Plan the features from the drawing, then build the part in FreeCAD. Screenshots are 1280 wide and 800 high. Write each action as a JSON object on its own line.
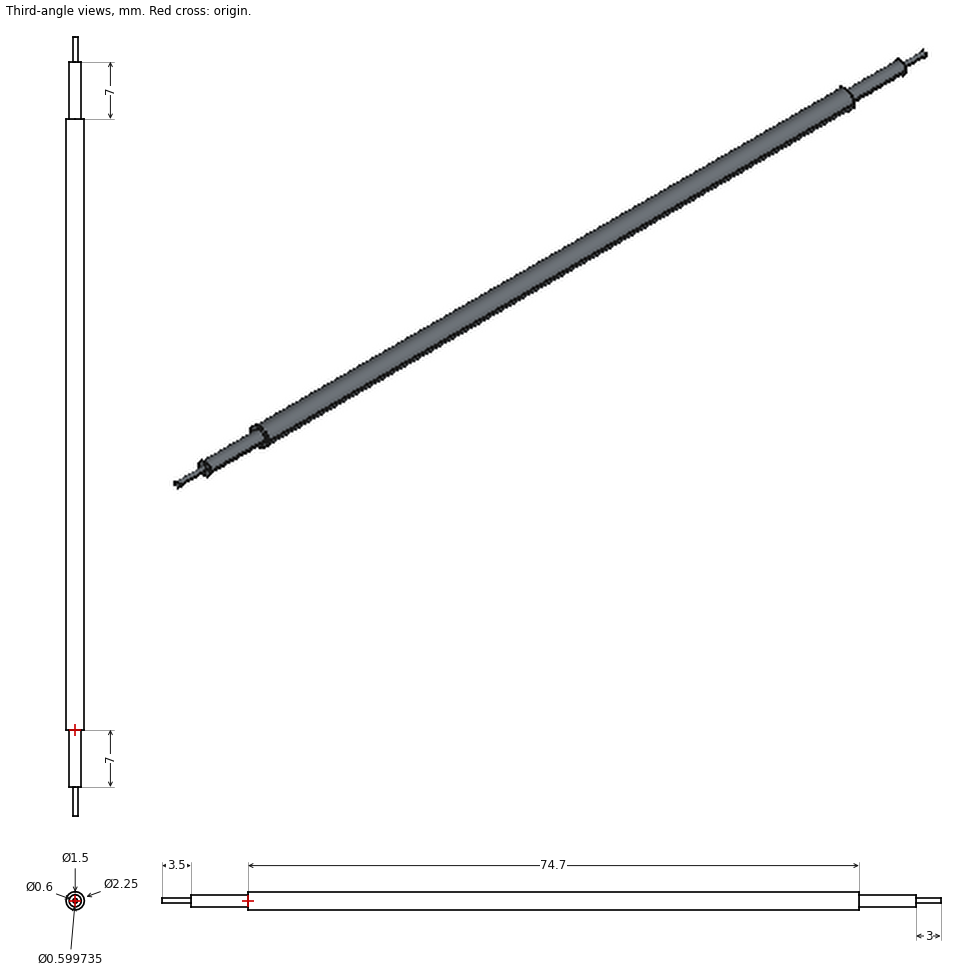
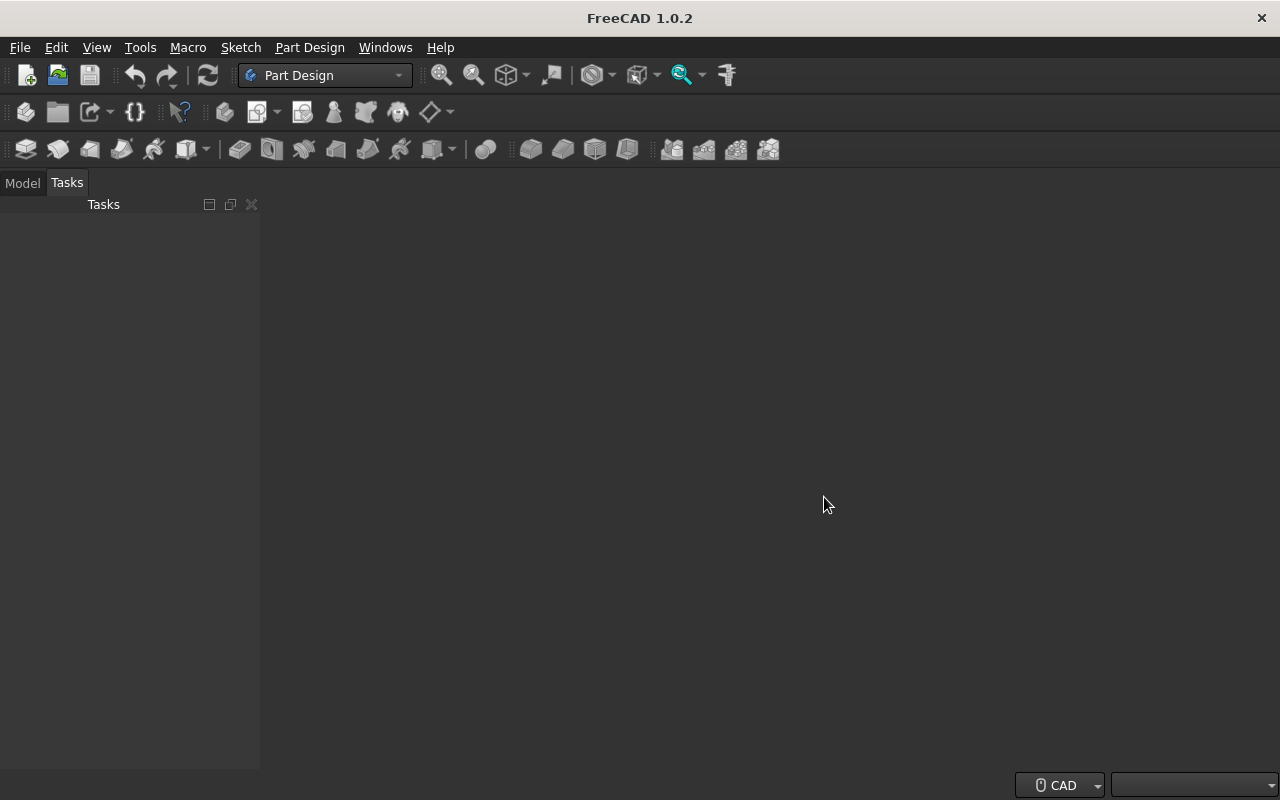
{"action": "left_click", "coordinate": [26, 76]}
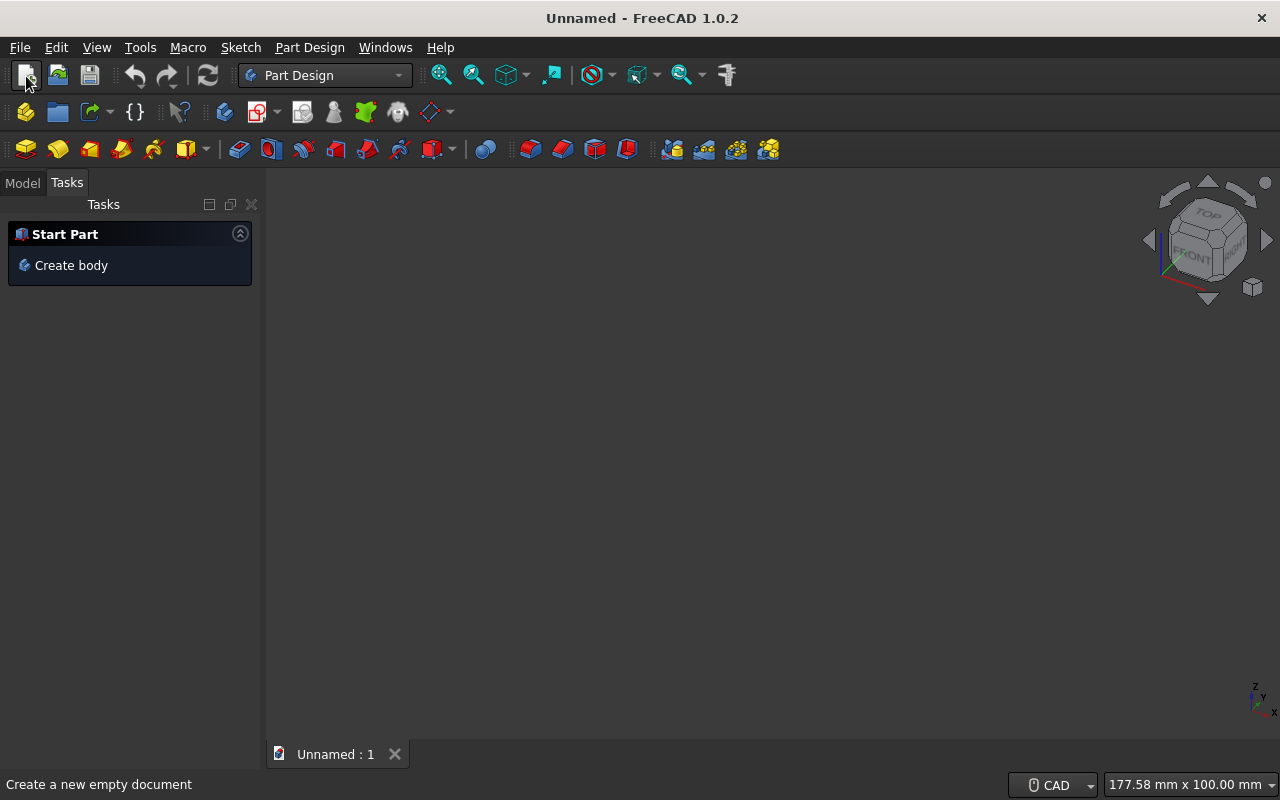
{"action": "left_click", "coordinate": [258, 112]}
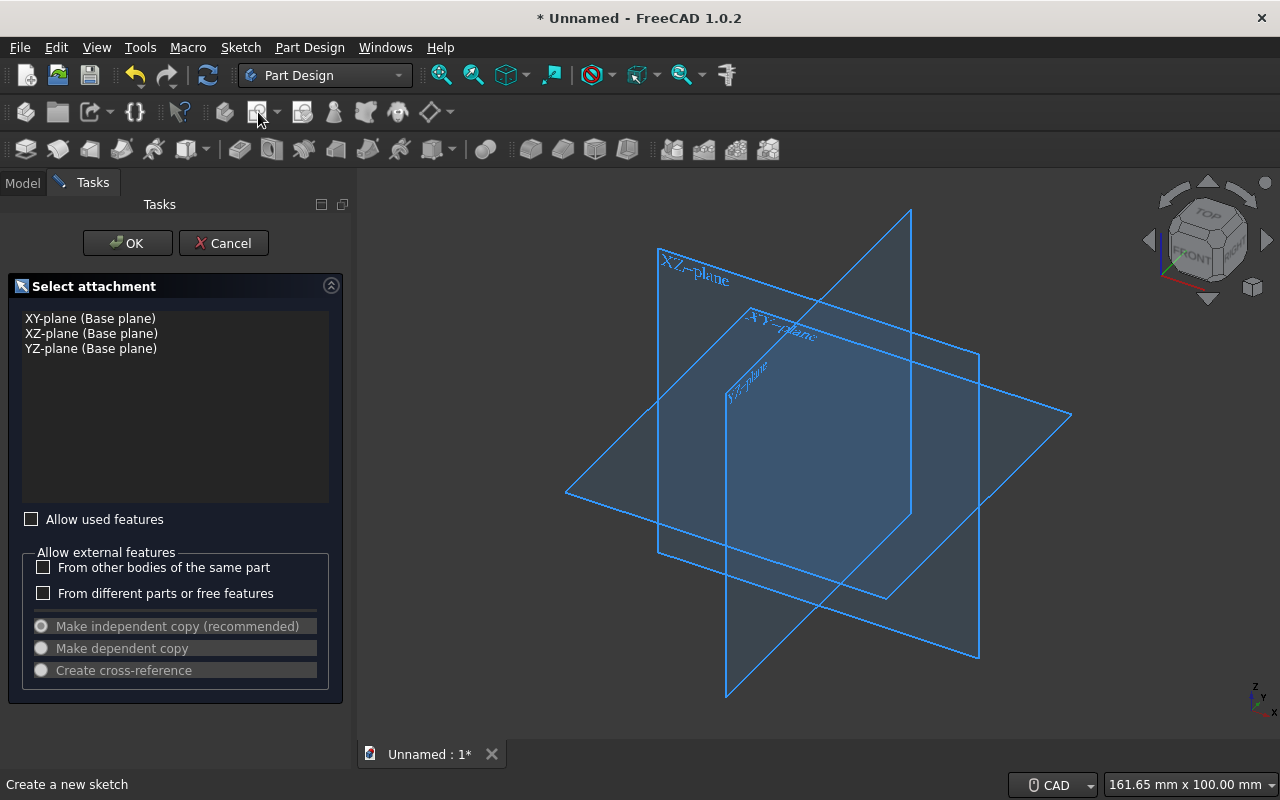
{"action": "left_click", "coordinate": [82, 334]}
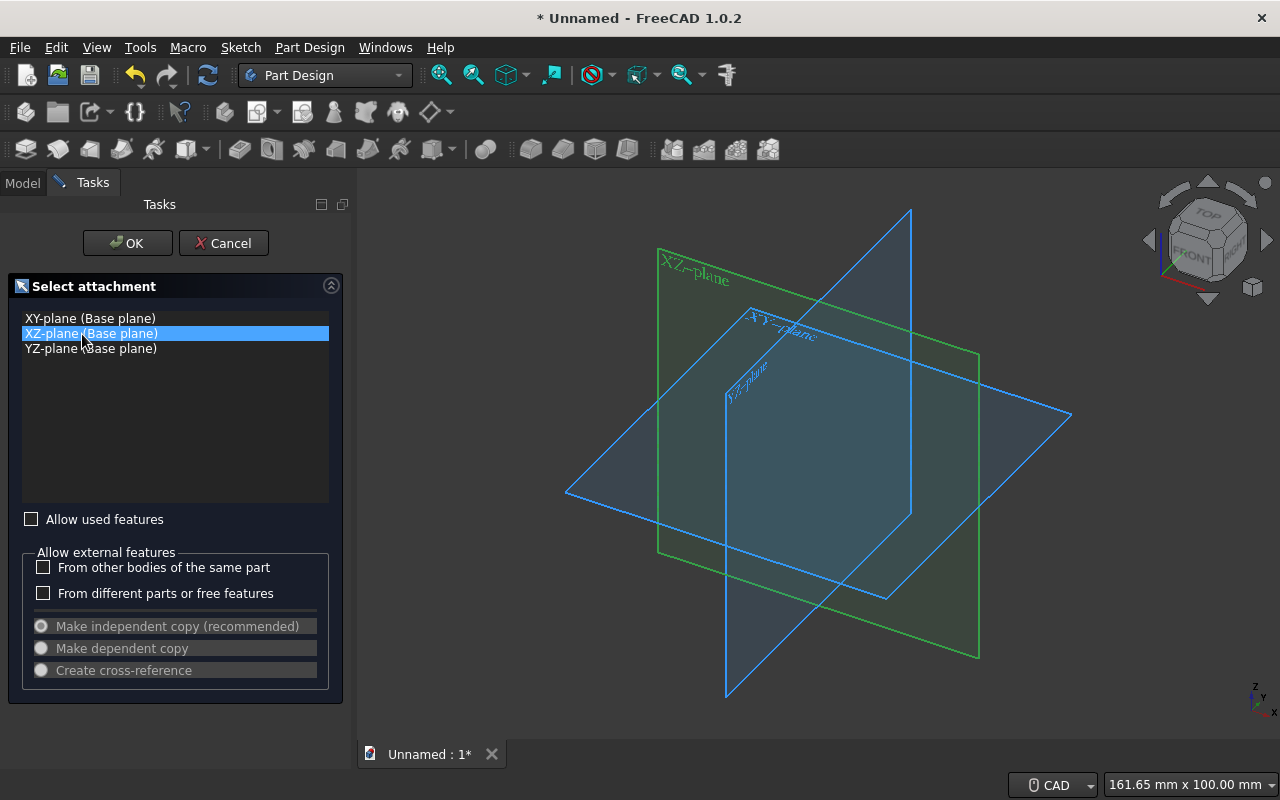
{"action": "left_click", "coordinate": [128, 243]}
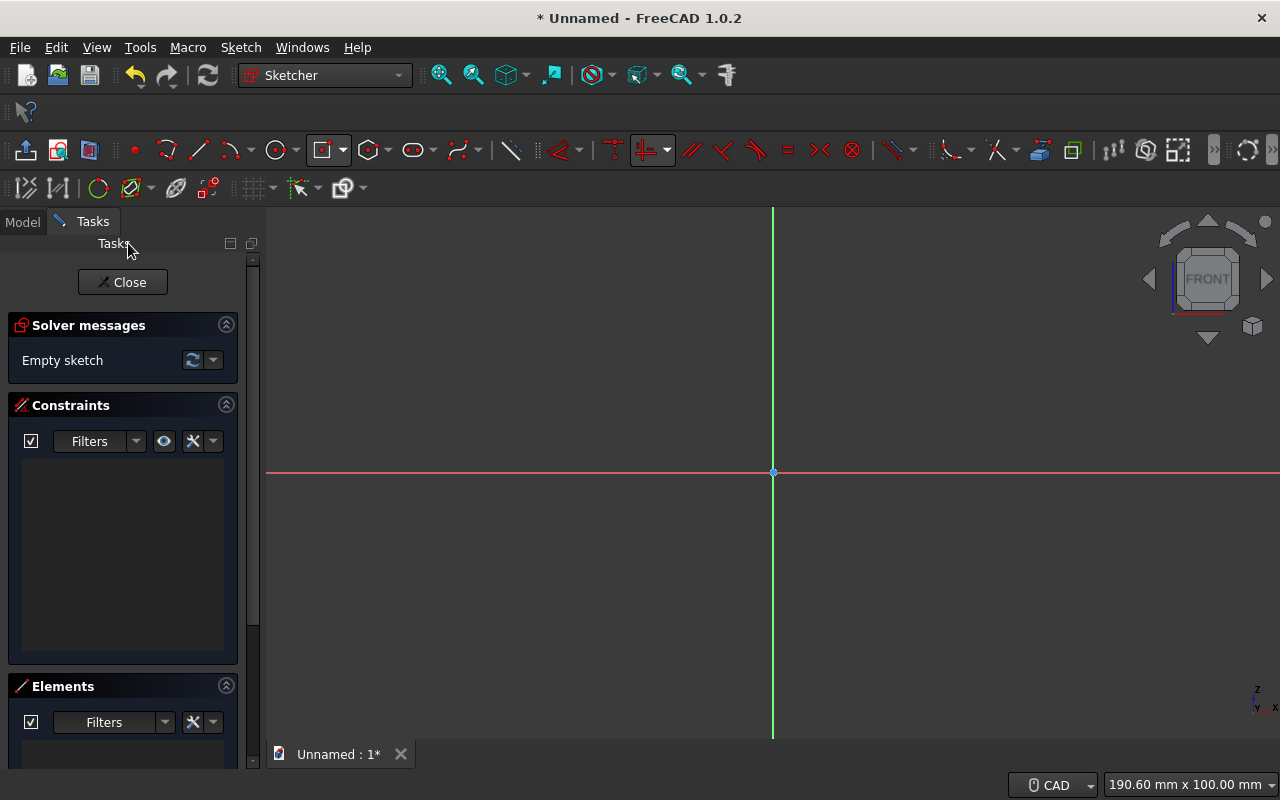
{"action": "scroll", "coordinate": [777, 473], "scroll_direction": "up", "scroll_amount": 15}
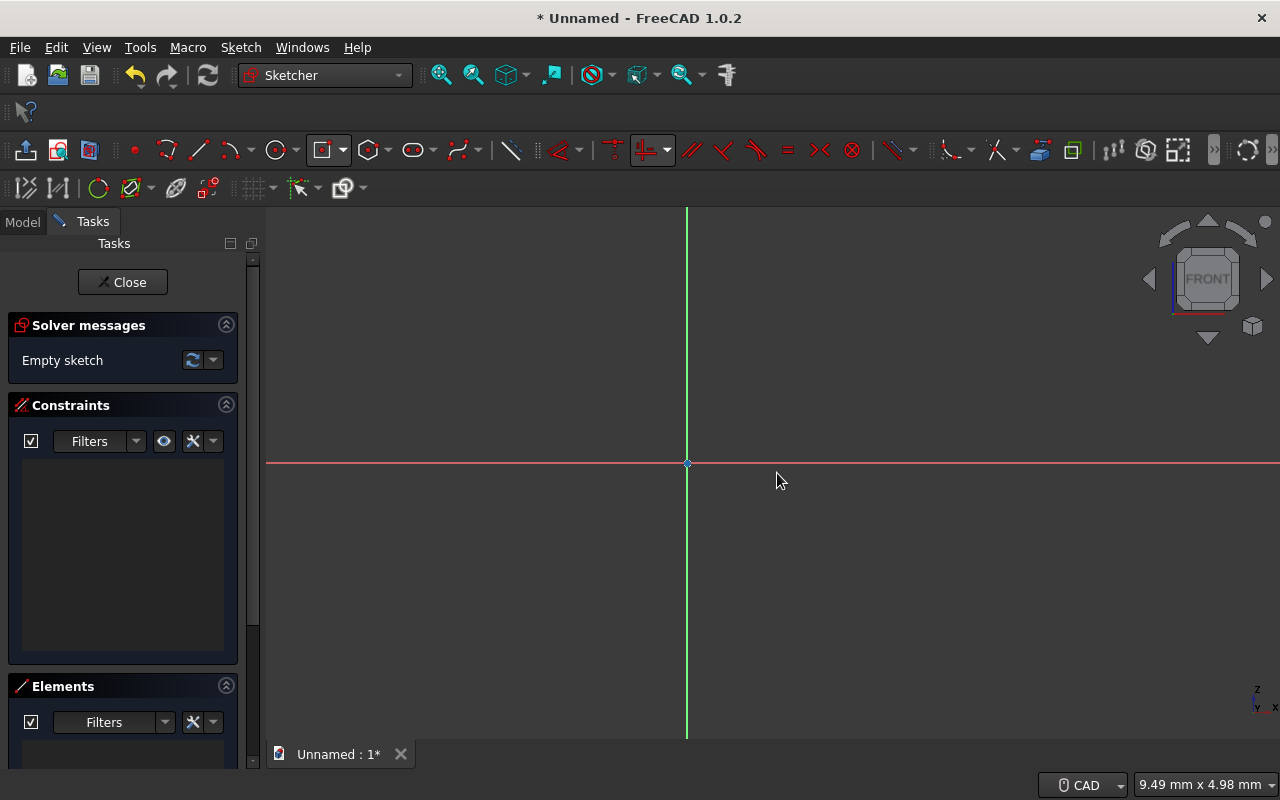
{"action": "scroll", "coordinate": [652, 444], "scroll_direction": "up", "scroll_amount": 2}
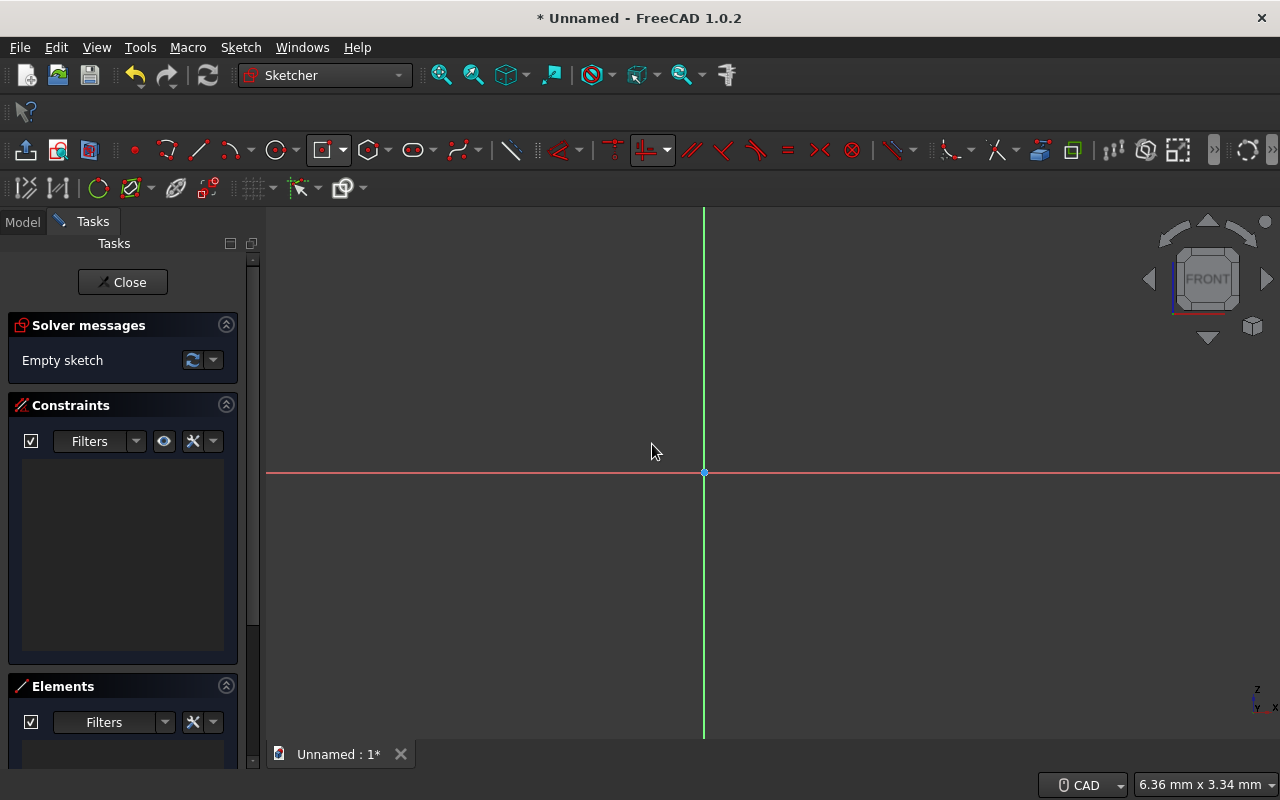
{"action": "left_click", "coordinate": [276, 150]}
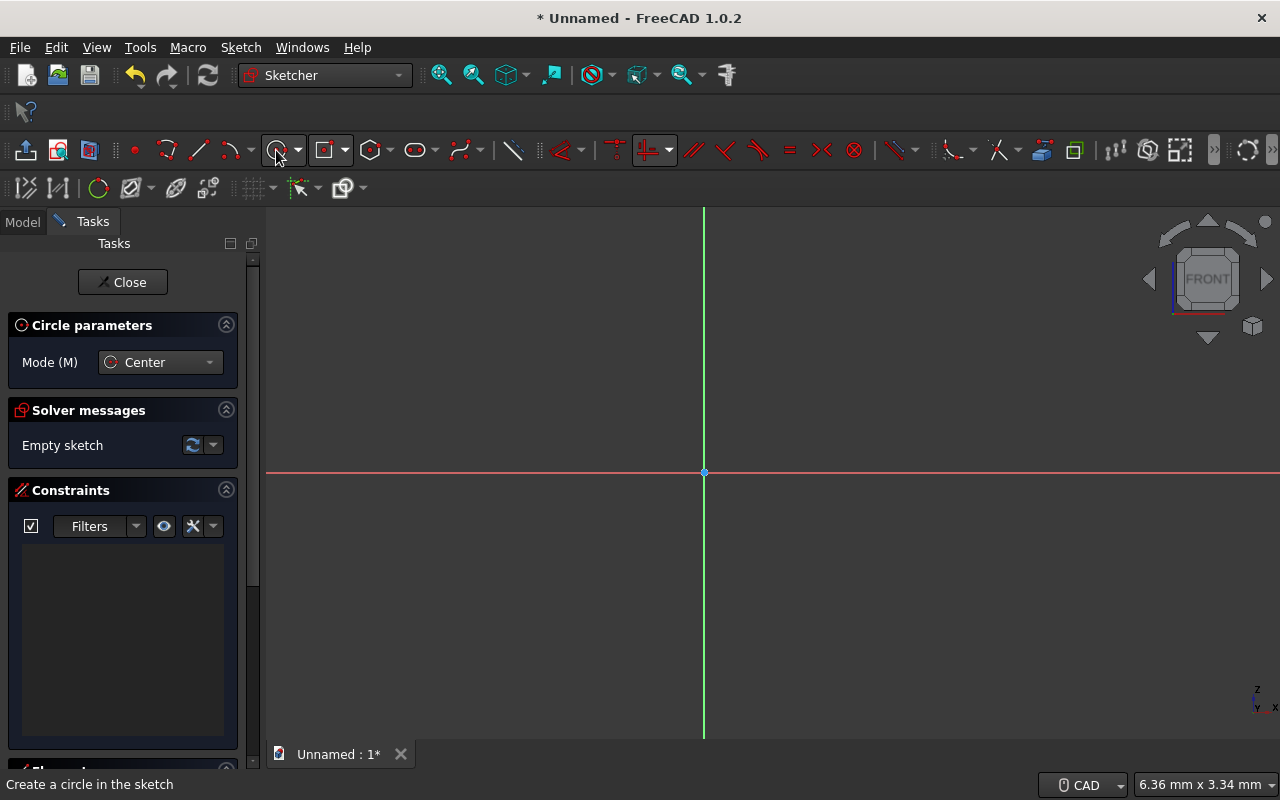
{"action": "left_click", "coordinate": [704, 473]}
{"action": "mouse_move", "coordinate": [831, 346]}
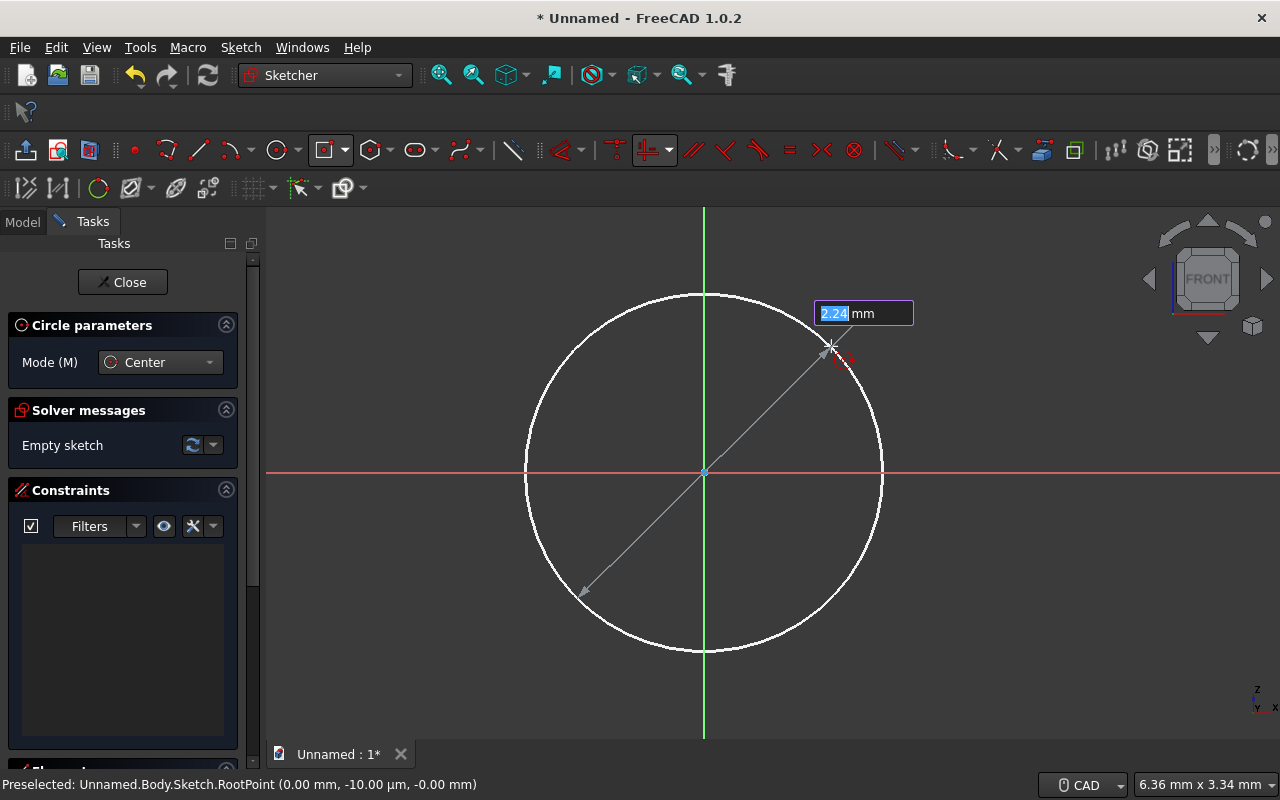
{"action": "type", "text": "2.25"}
{"action": "key", "text": "Return"}
{"action": "key", "text": "Escape"}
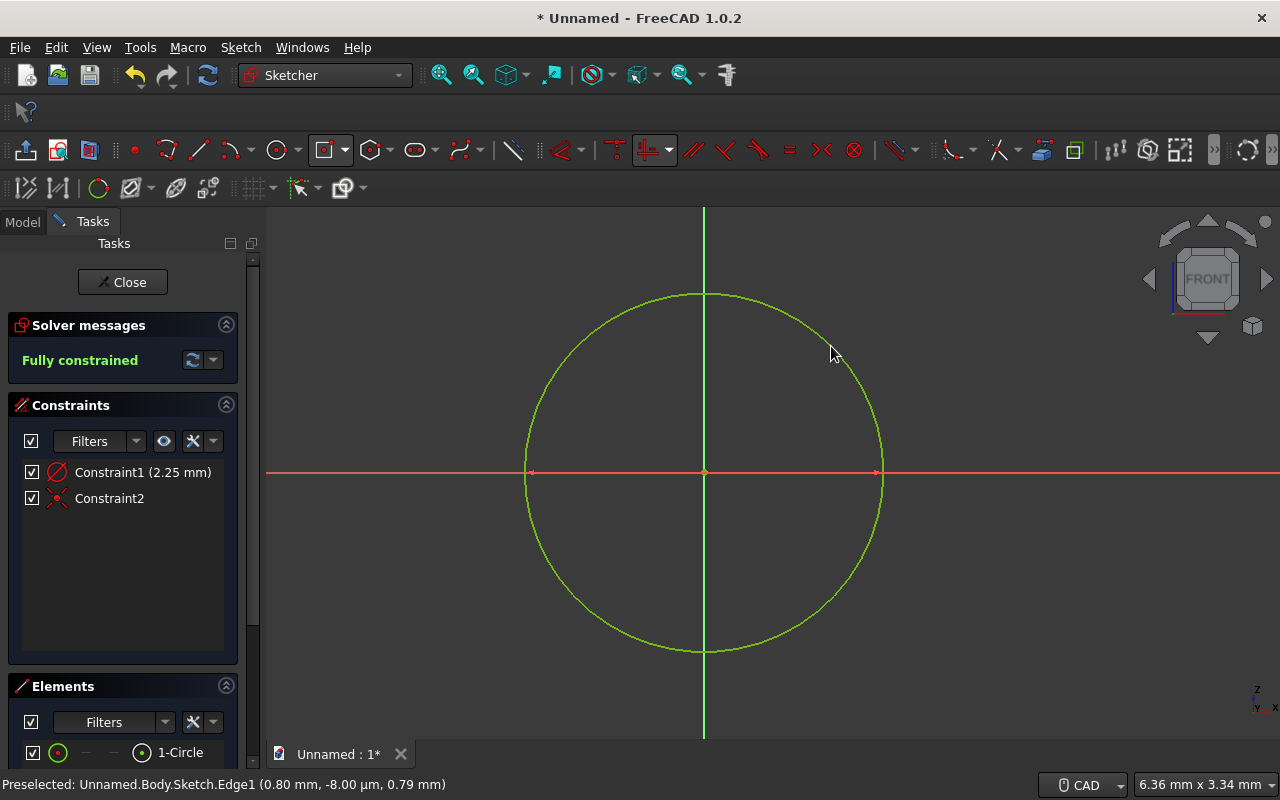
{"action": "left_click", "coordinate": [123, 282]}